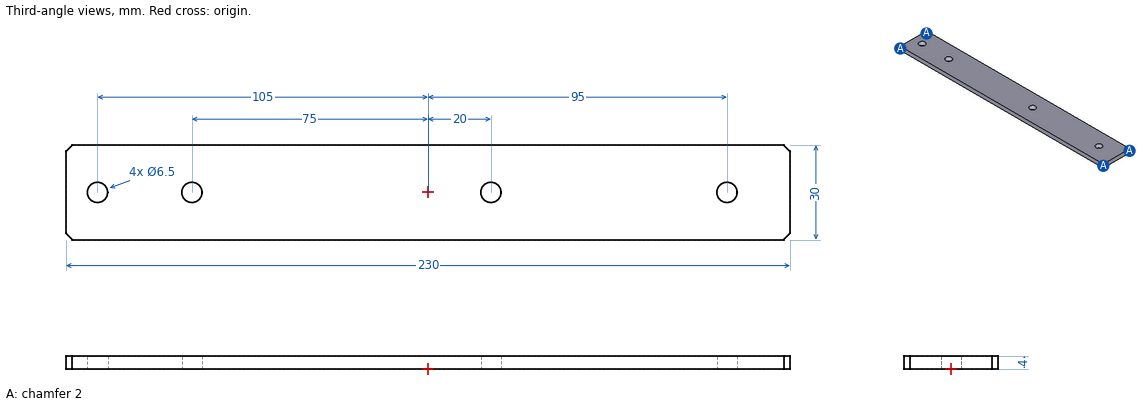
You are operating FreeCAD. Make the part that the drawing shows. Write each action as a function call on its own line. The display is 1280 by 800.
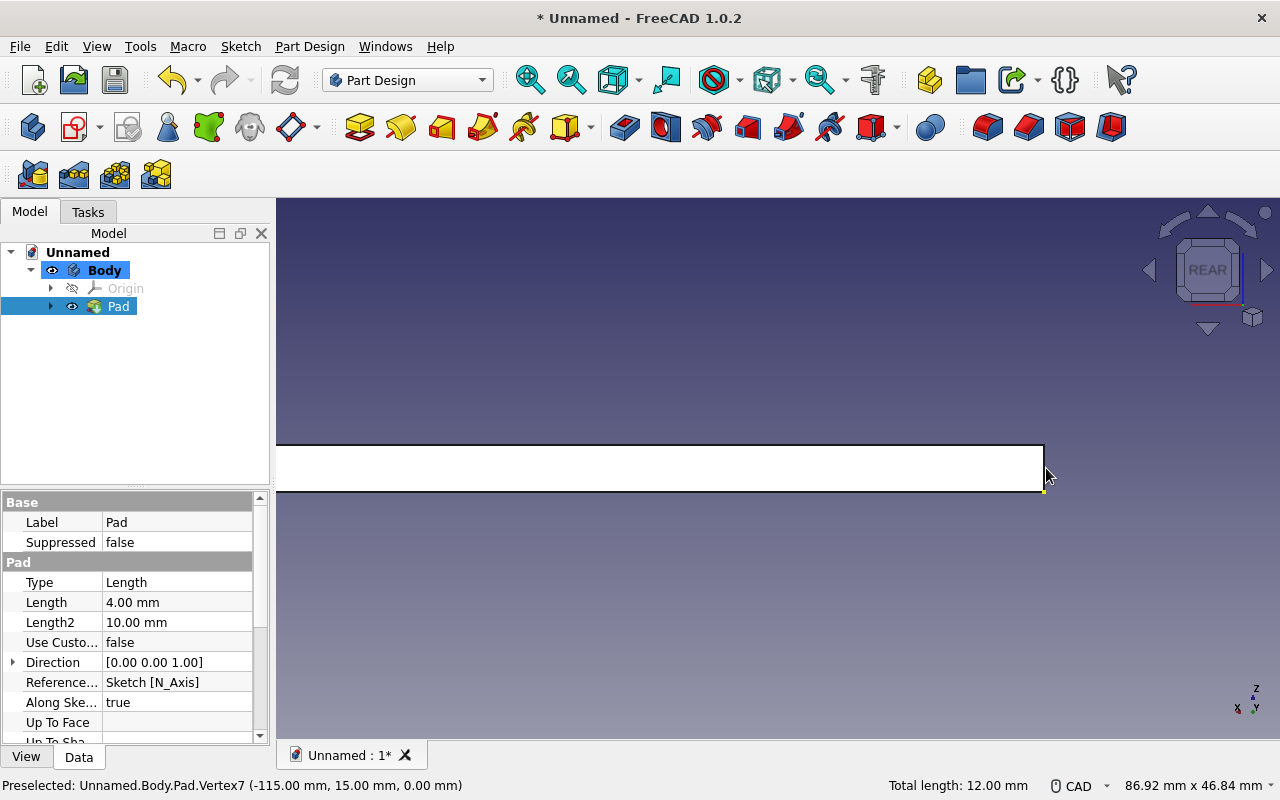
click(1044, 468, ctrl)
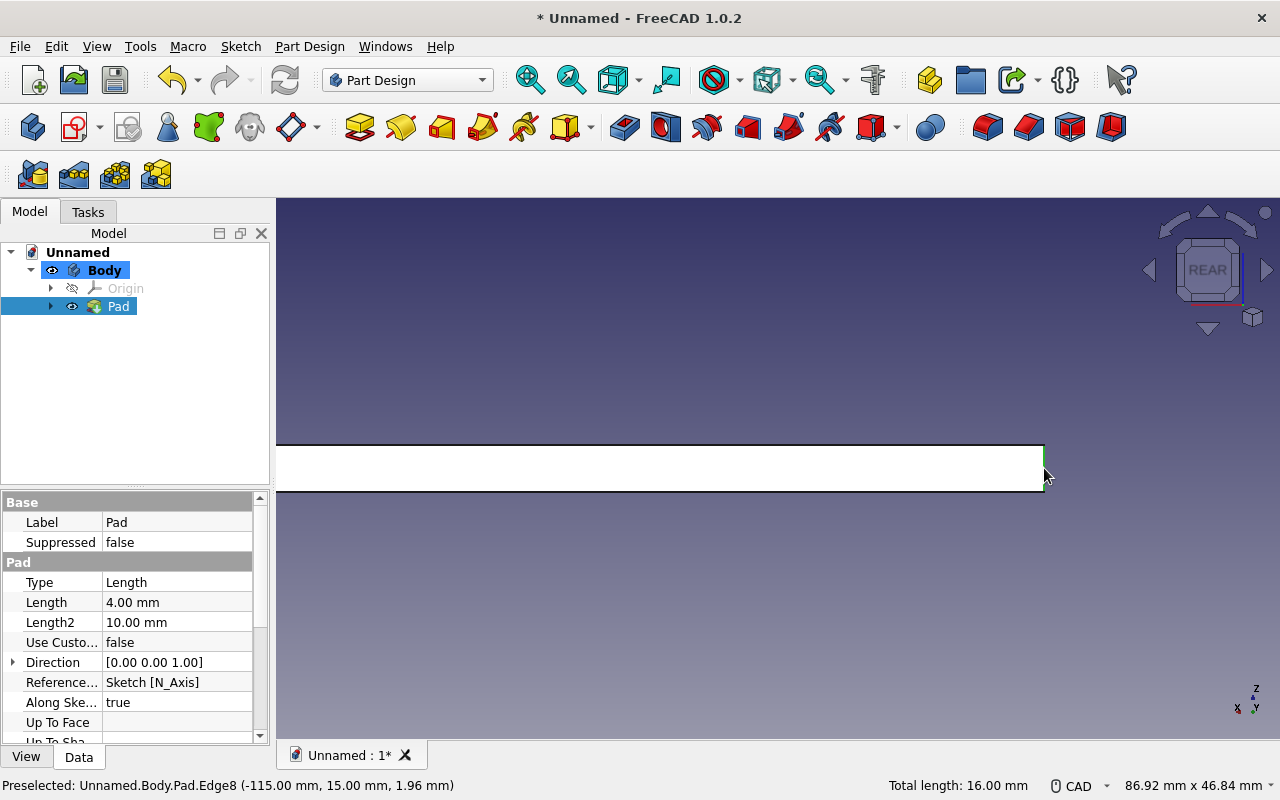
click(1029, 128)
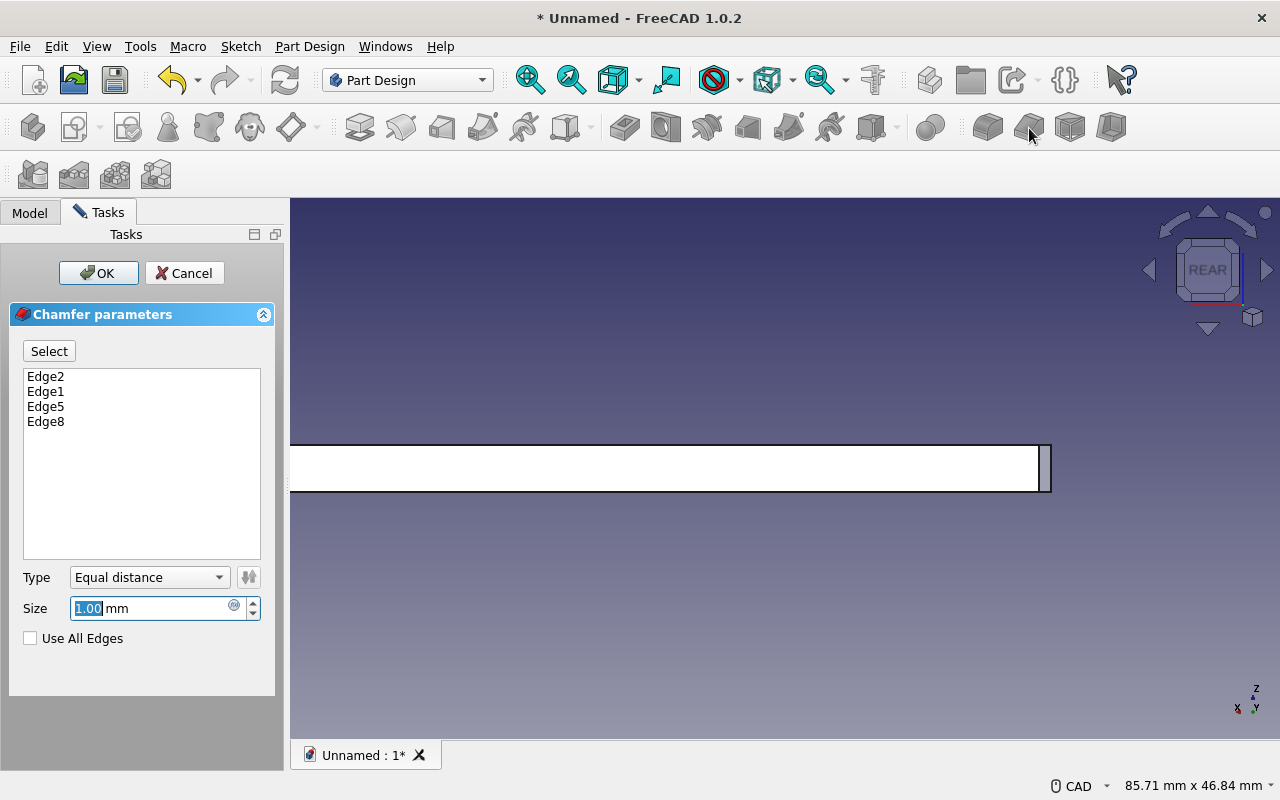
text(2)
key(Tab)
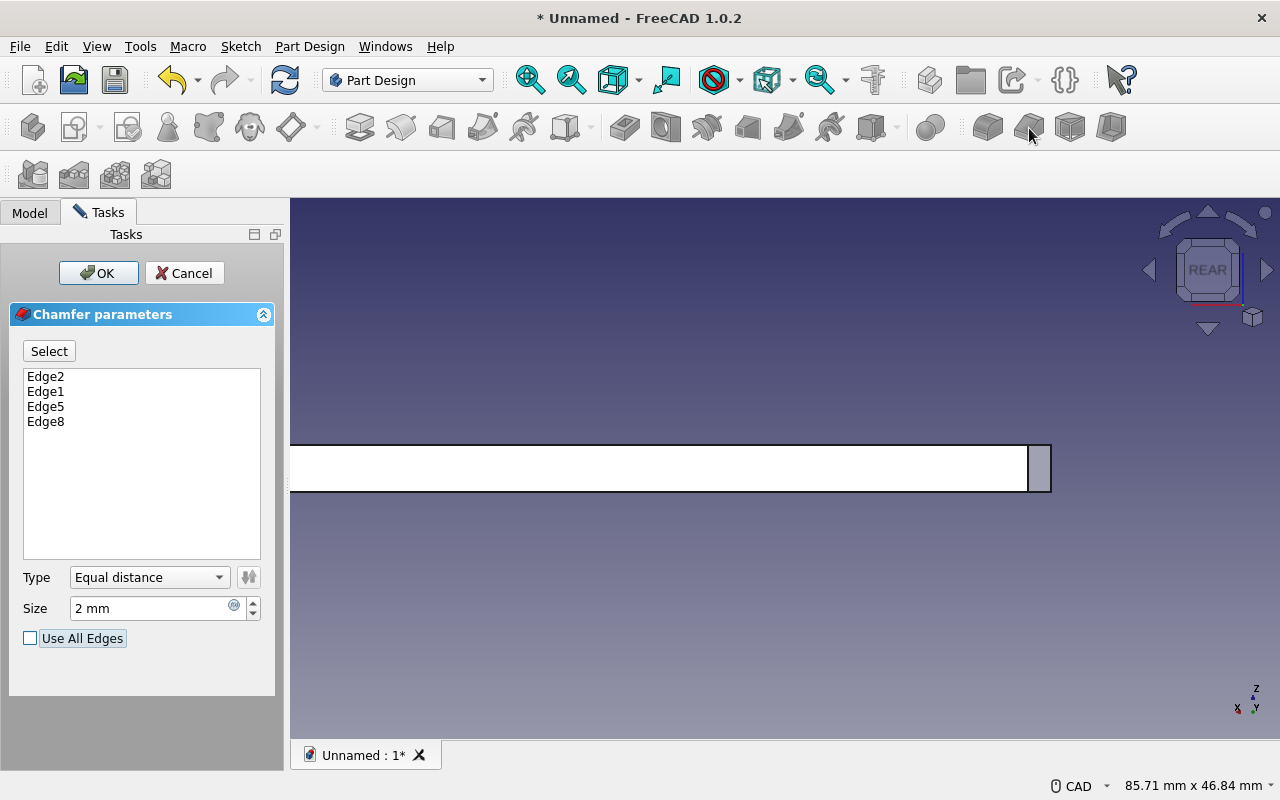
click(99, 273)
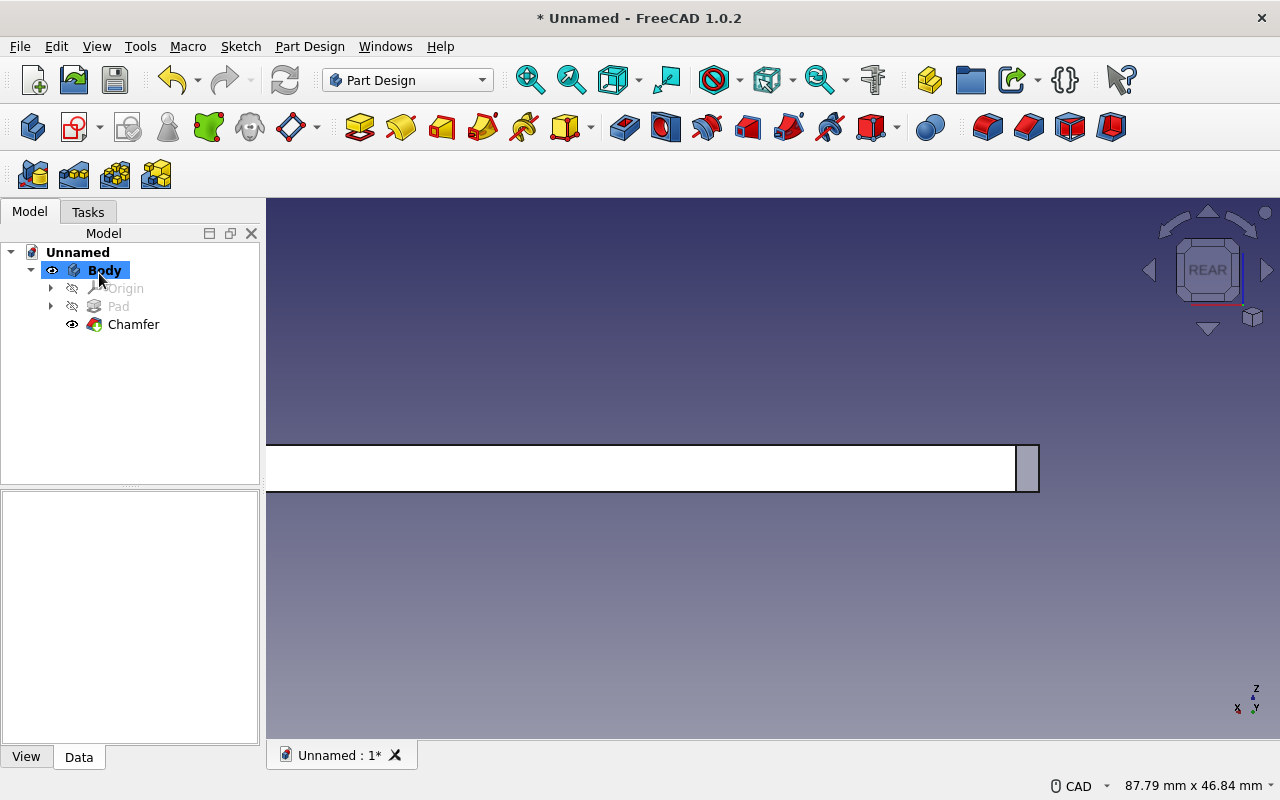
key(0)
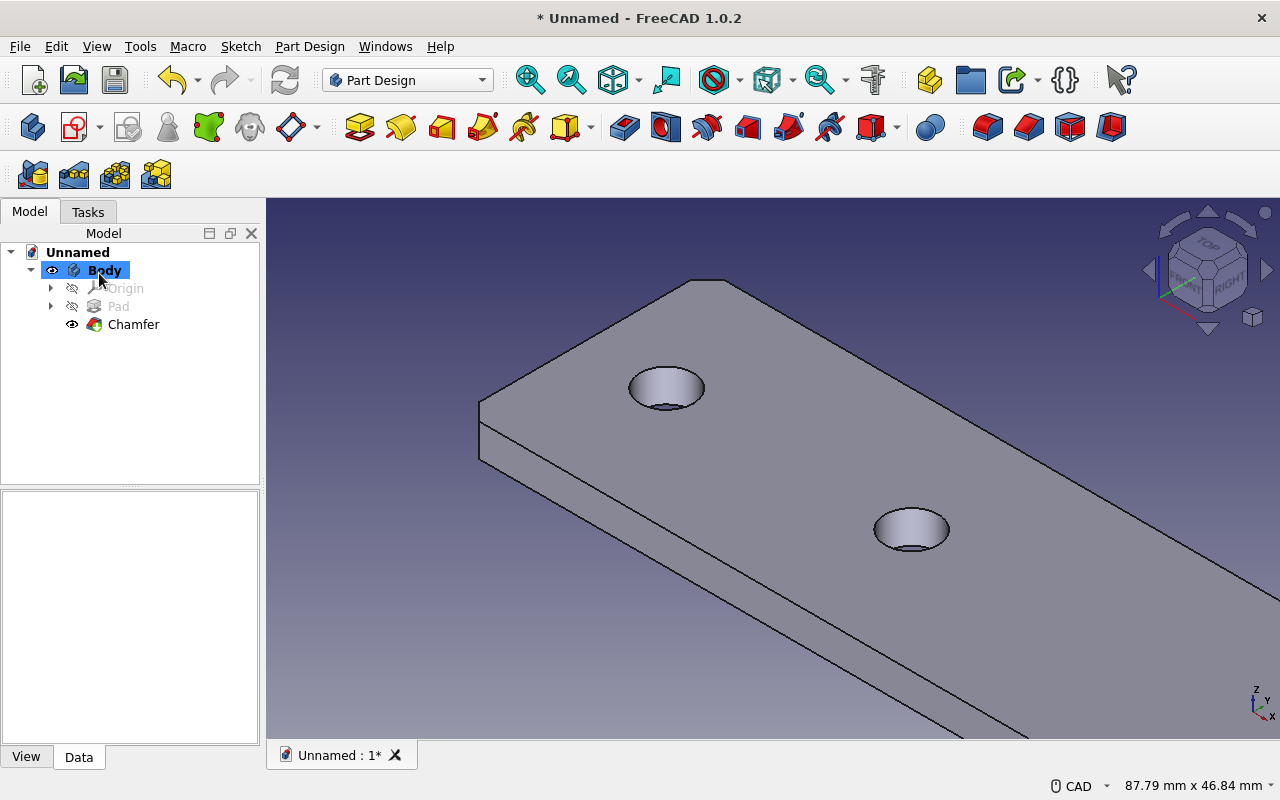
click(531, 80)